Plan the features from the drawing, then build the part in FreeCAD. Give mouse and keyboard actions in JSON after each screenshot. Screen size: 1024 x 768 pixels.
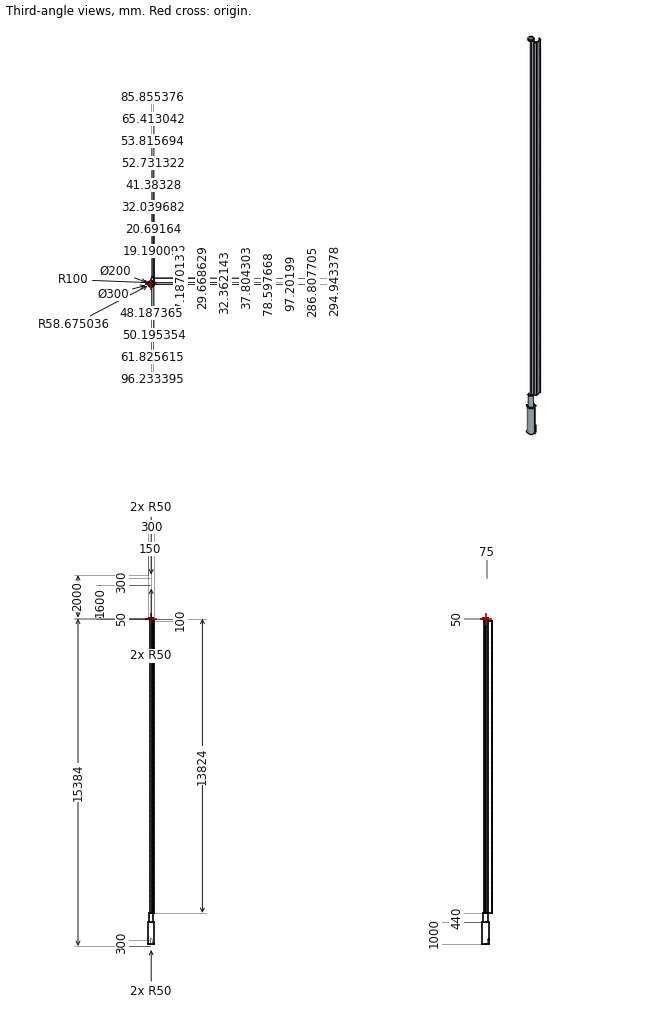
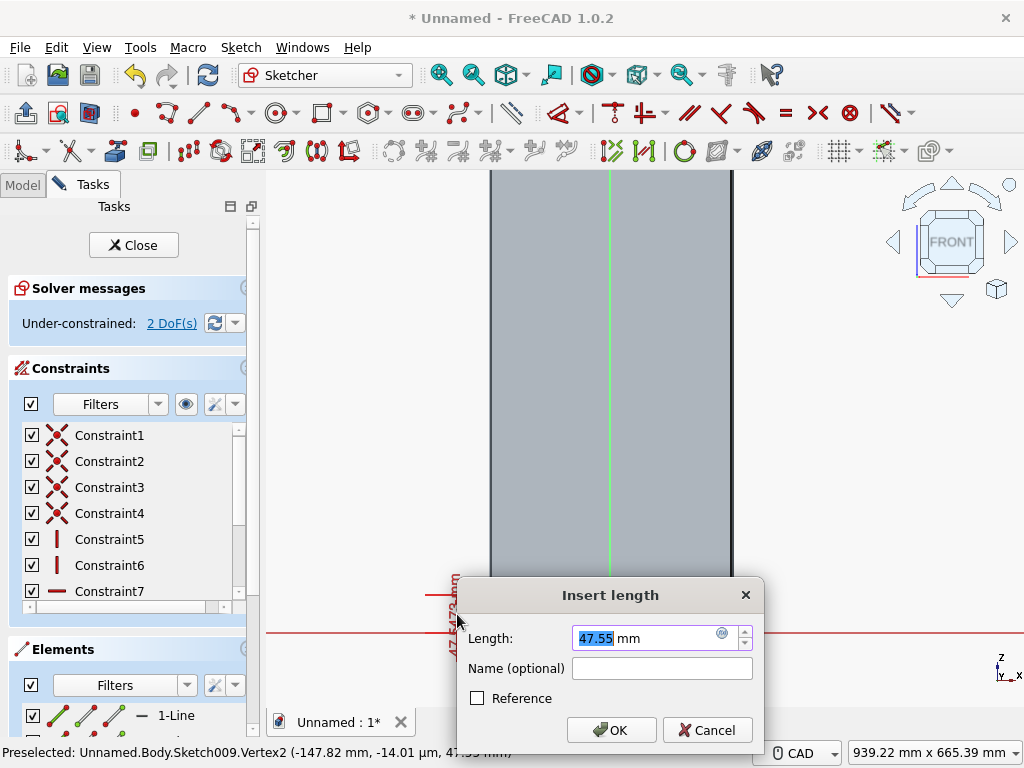
{"action": "type", "text": "50"}
{"action": "key", "text": "Return"}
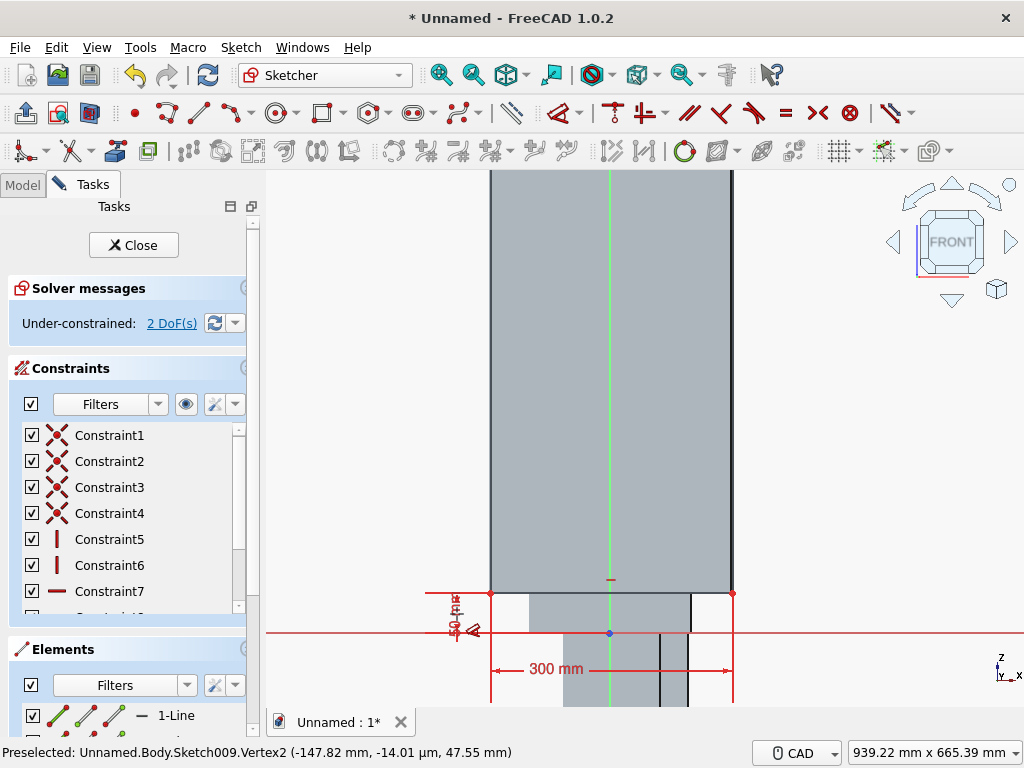
{"action": "scroll", "coordinate": [568, 598], "scroll_direction": "down", "scroll_amount": 8}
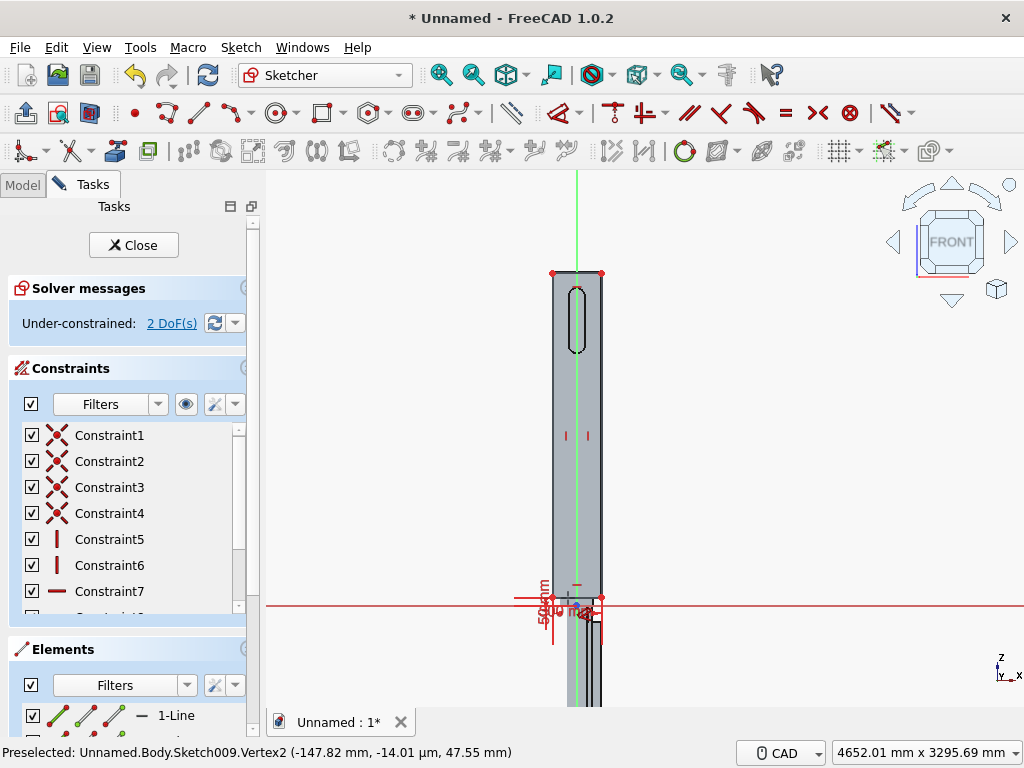
{"action": "left_click", "coordinate": [553, 533]}
{"action": "left_click", "coordinate": [519, 435]}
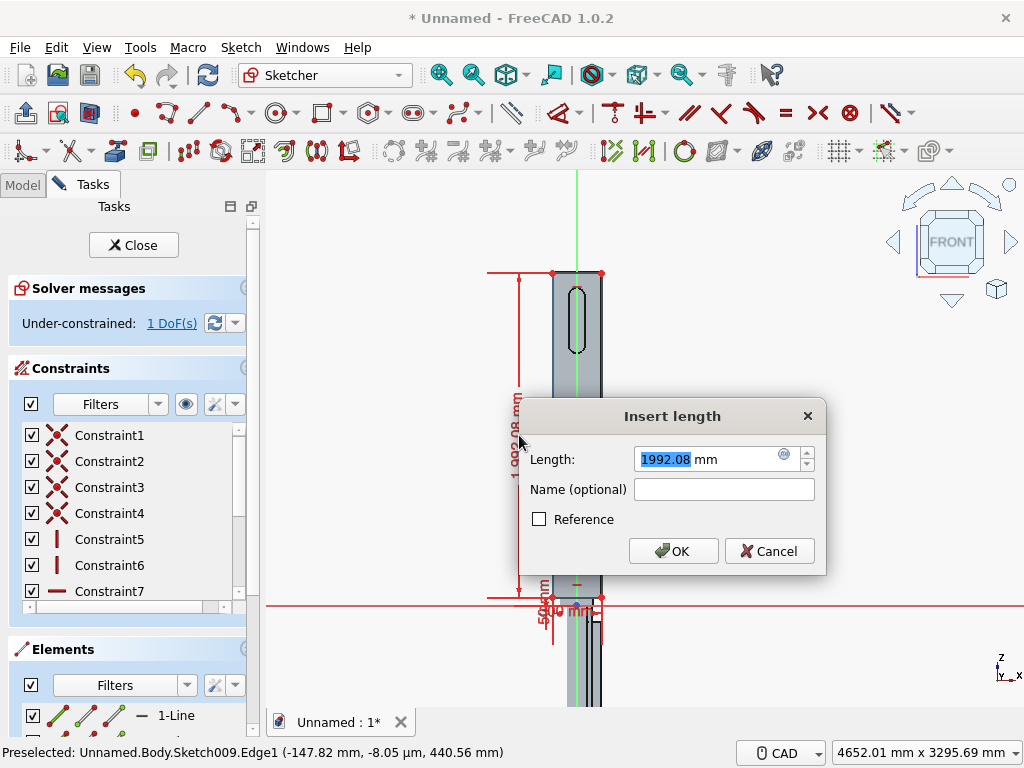
{"action": "type", "text": "2000"}
{"action": "key", "text": "Return"}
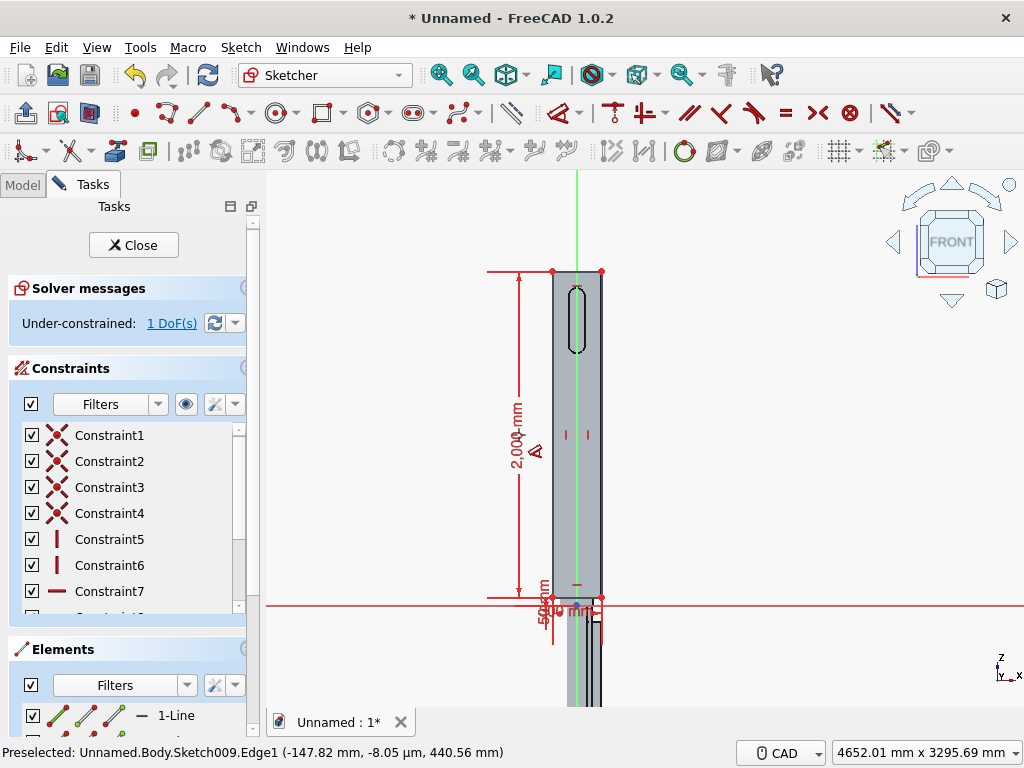
{"action": "scroll", "coordinate": [553, 272], "scroll_direction": "up", "scroll_amount": 3}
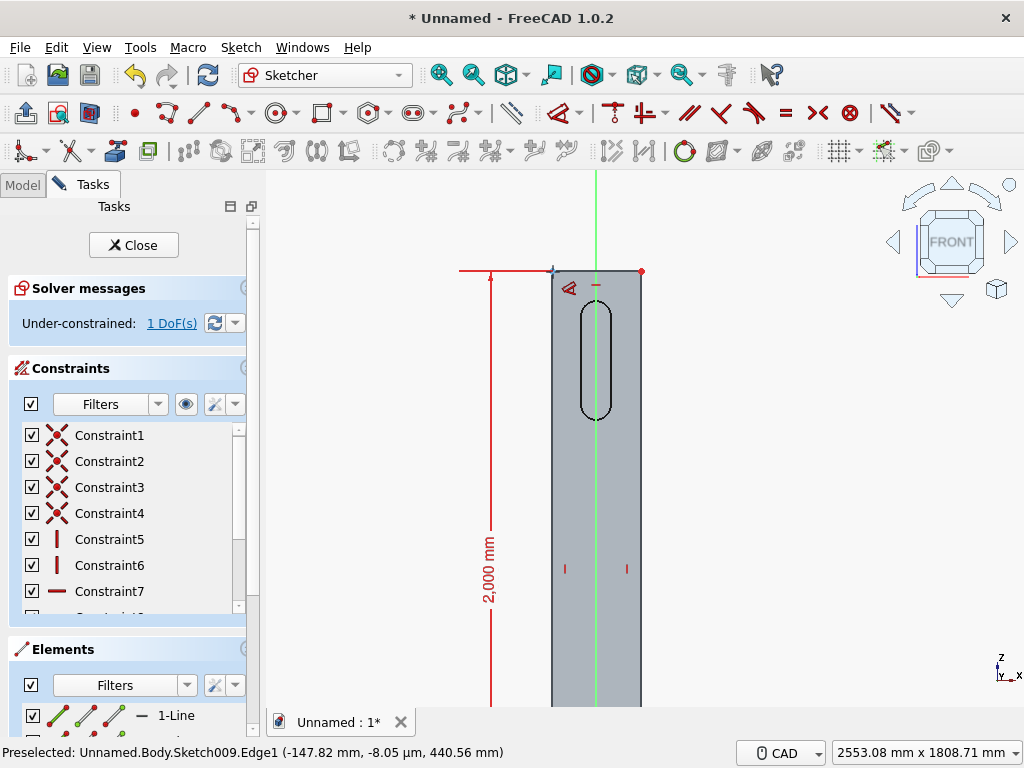
{"action": "left_click", "coordinate": [552, 271]}
{"action": "left_click", "coordinate": [574, 237]}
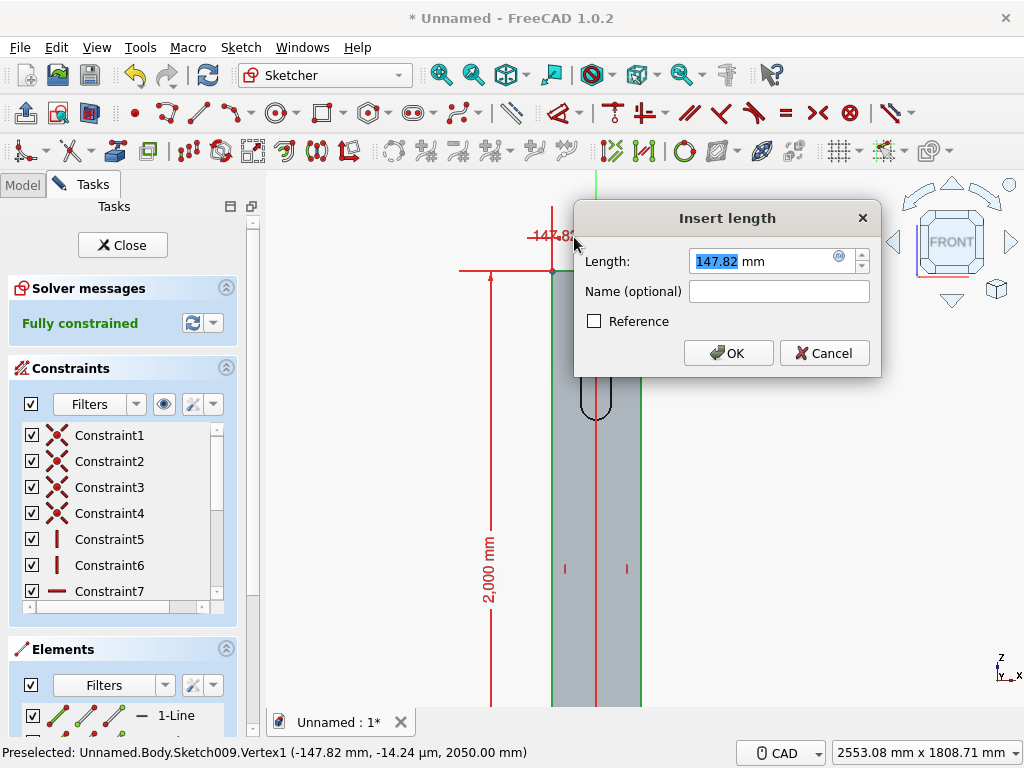
{"action": "type", "text": "150"}
{"action": "key", "text": "Return"}
{"action": "key", "text": "Escape"}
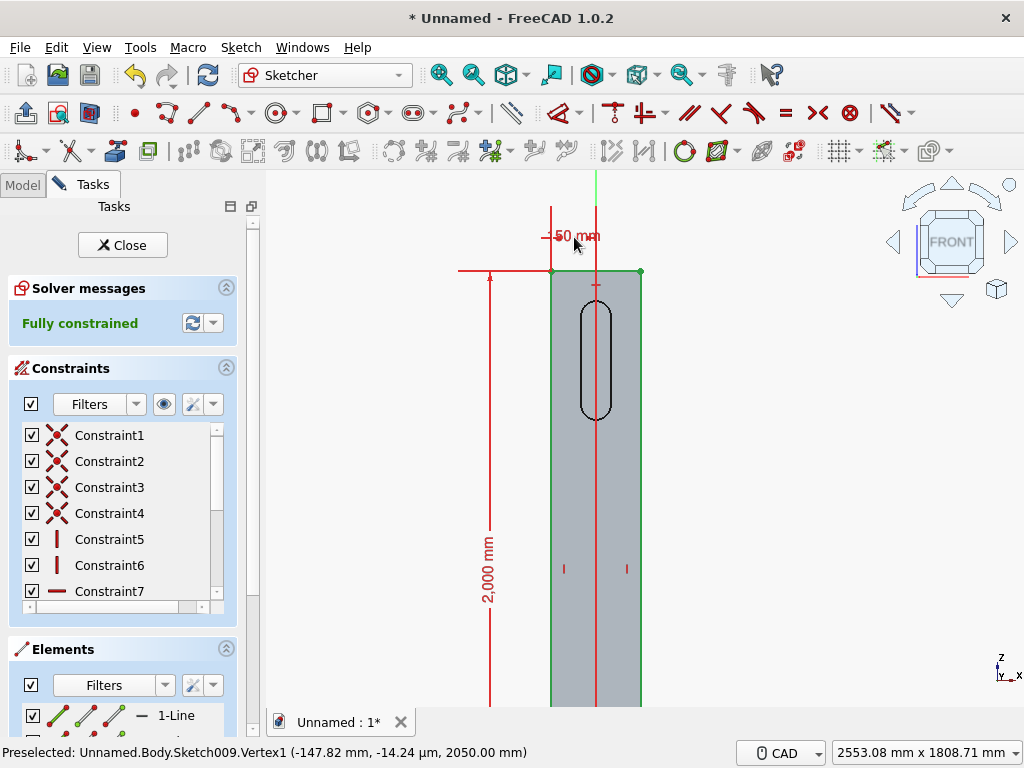
{"action": "left_click", "coordinate": [123, 245]}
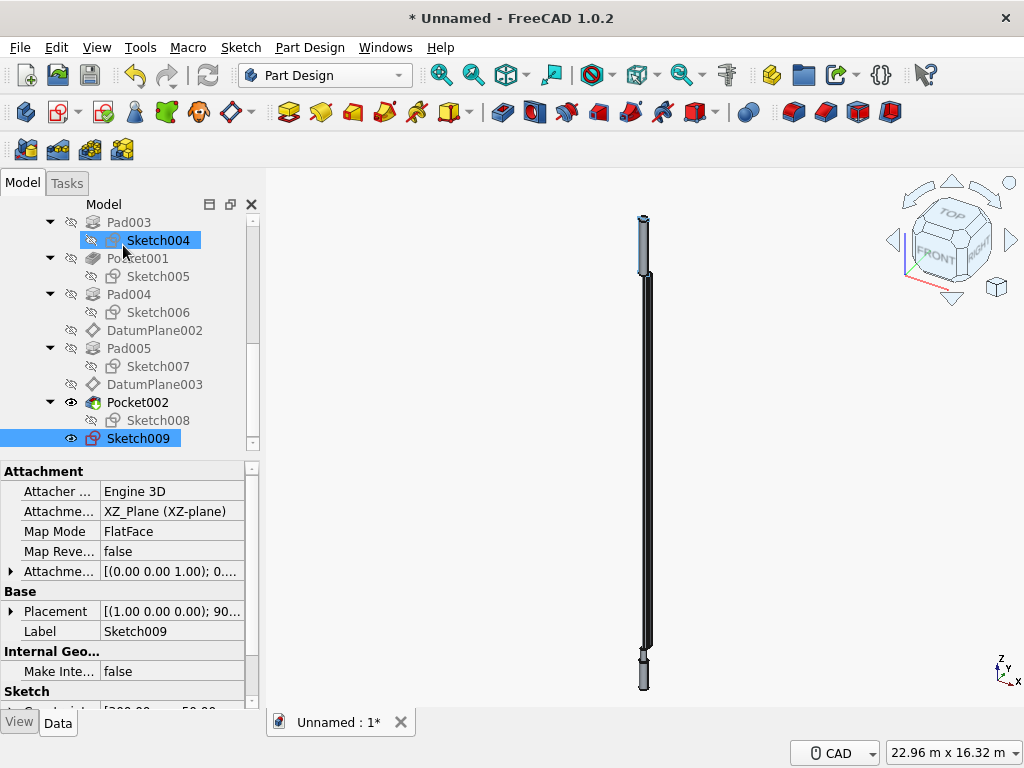
{"action": "left_click", "coordinate": [504, 112]}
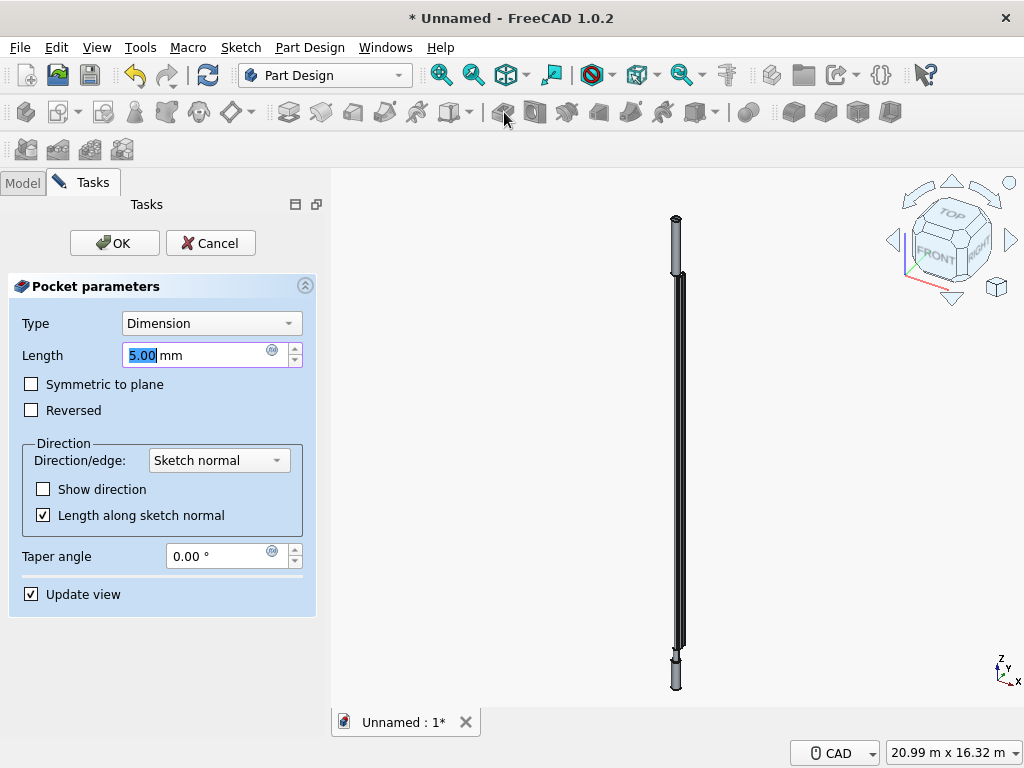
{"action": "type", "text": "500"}
{"action": "key", "text": "Tab"}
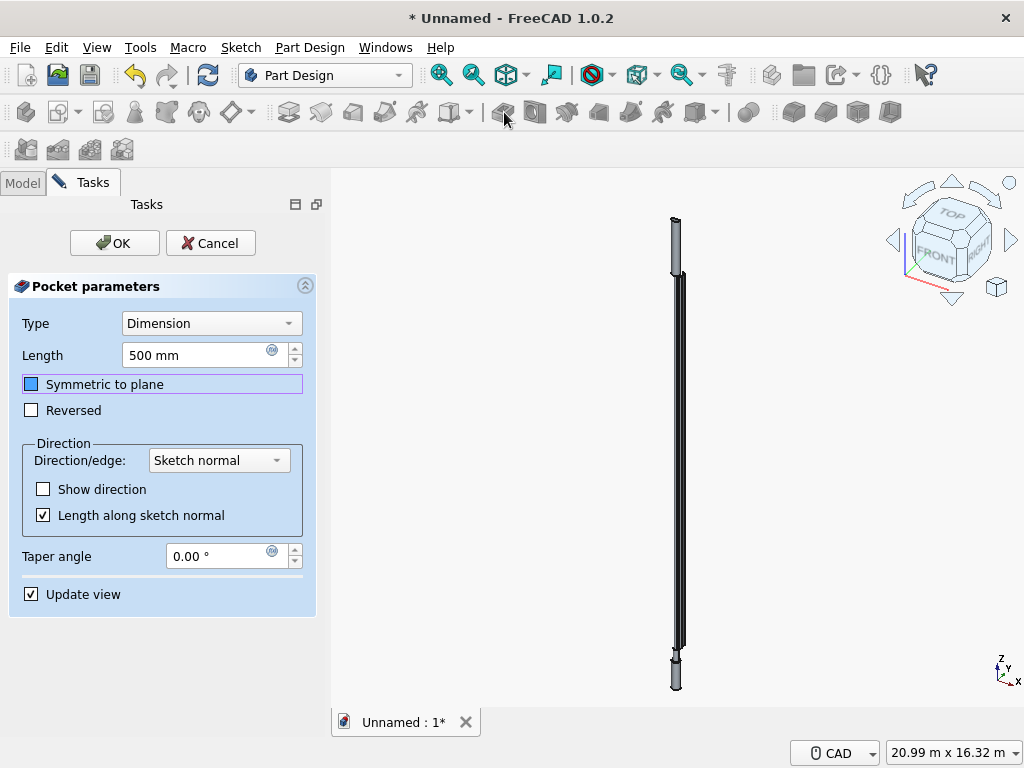
{"action": "left_click", "coordinate": [30, 384]}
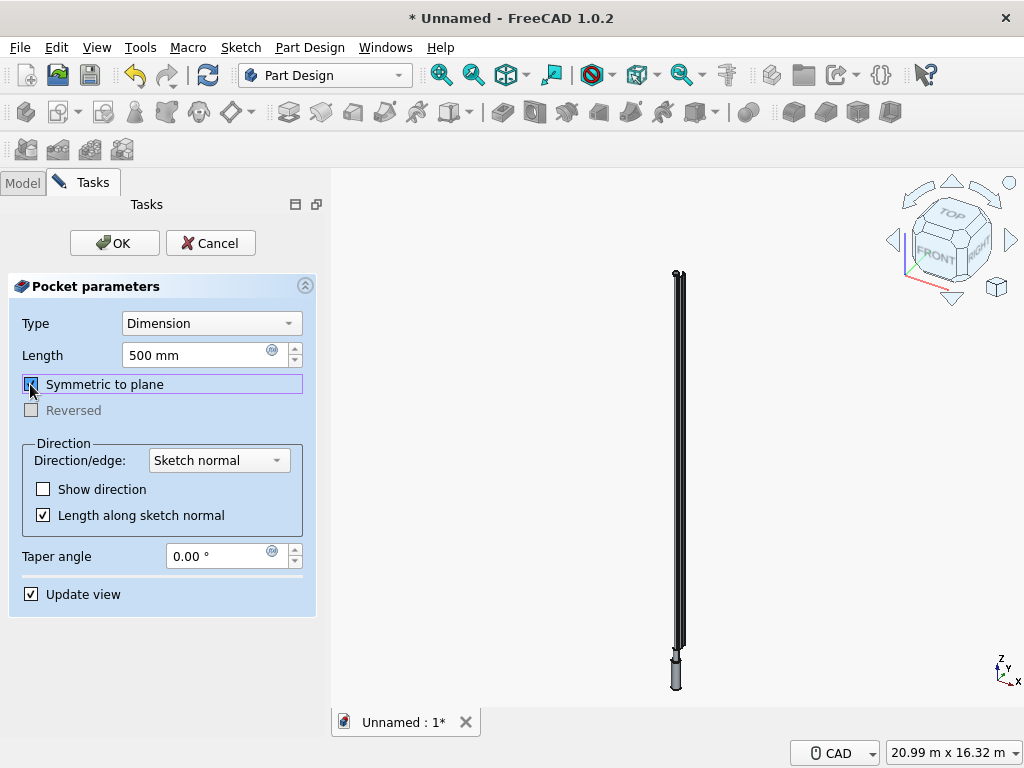
{"action": "left_click", "coordinate": [115, 243]}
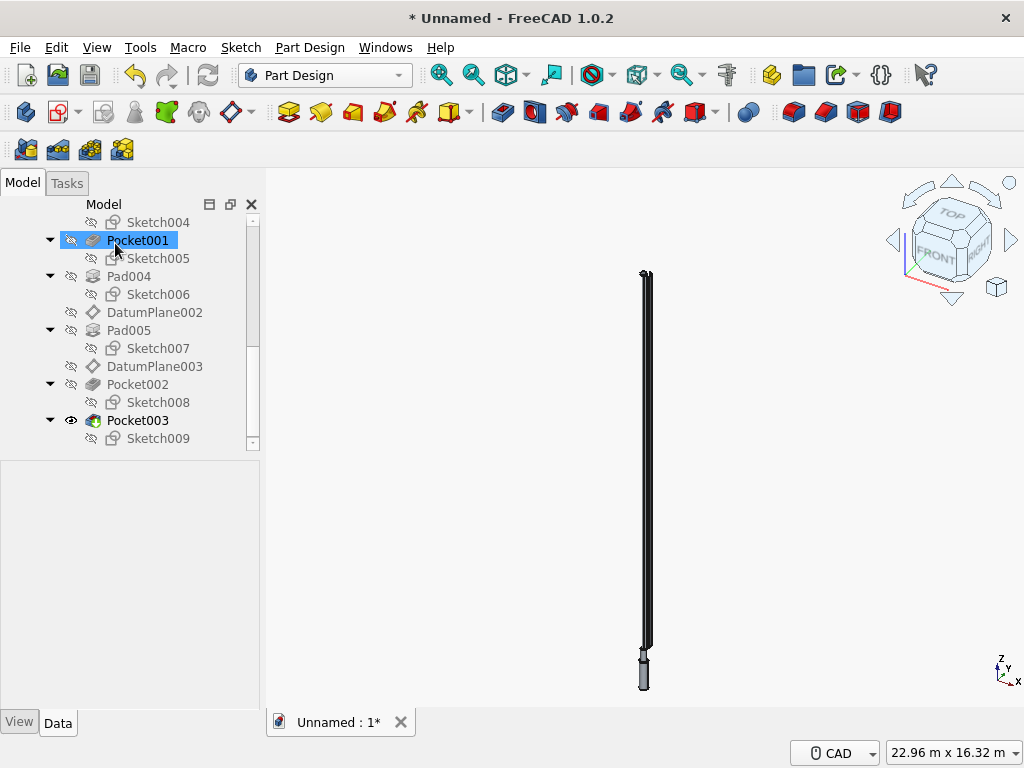
{"action": "key", "text": "0"}